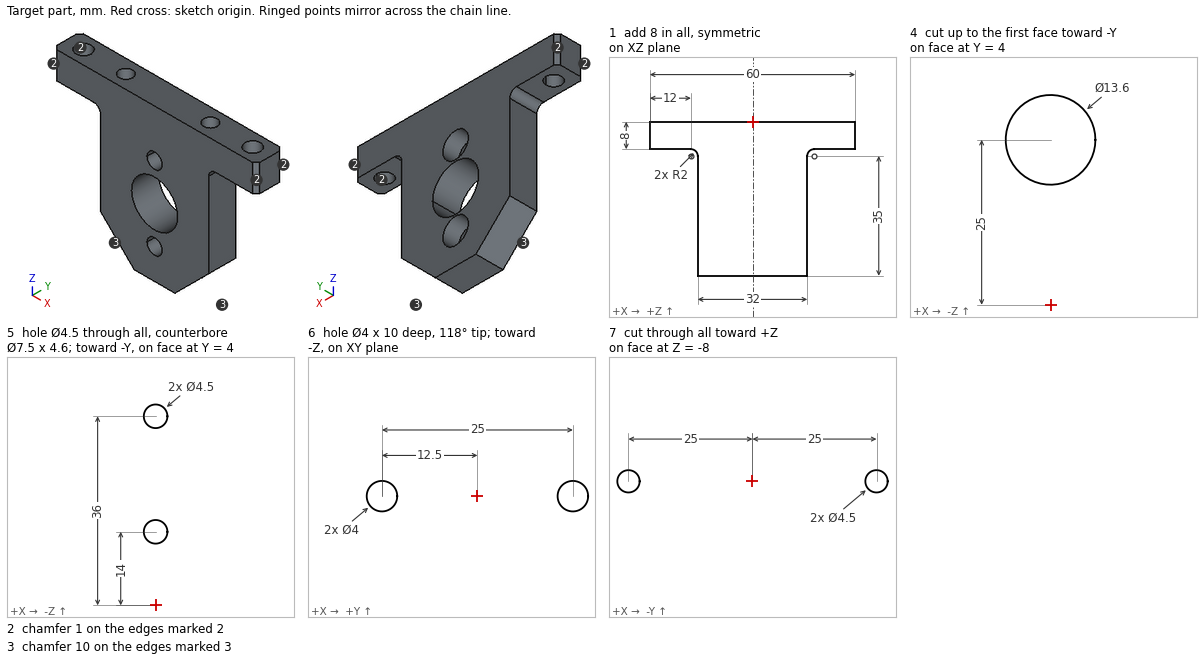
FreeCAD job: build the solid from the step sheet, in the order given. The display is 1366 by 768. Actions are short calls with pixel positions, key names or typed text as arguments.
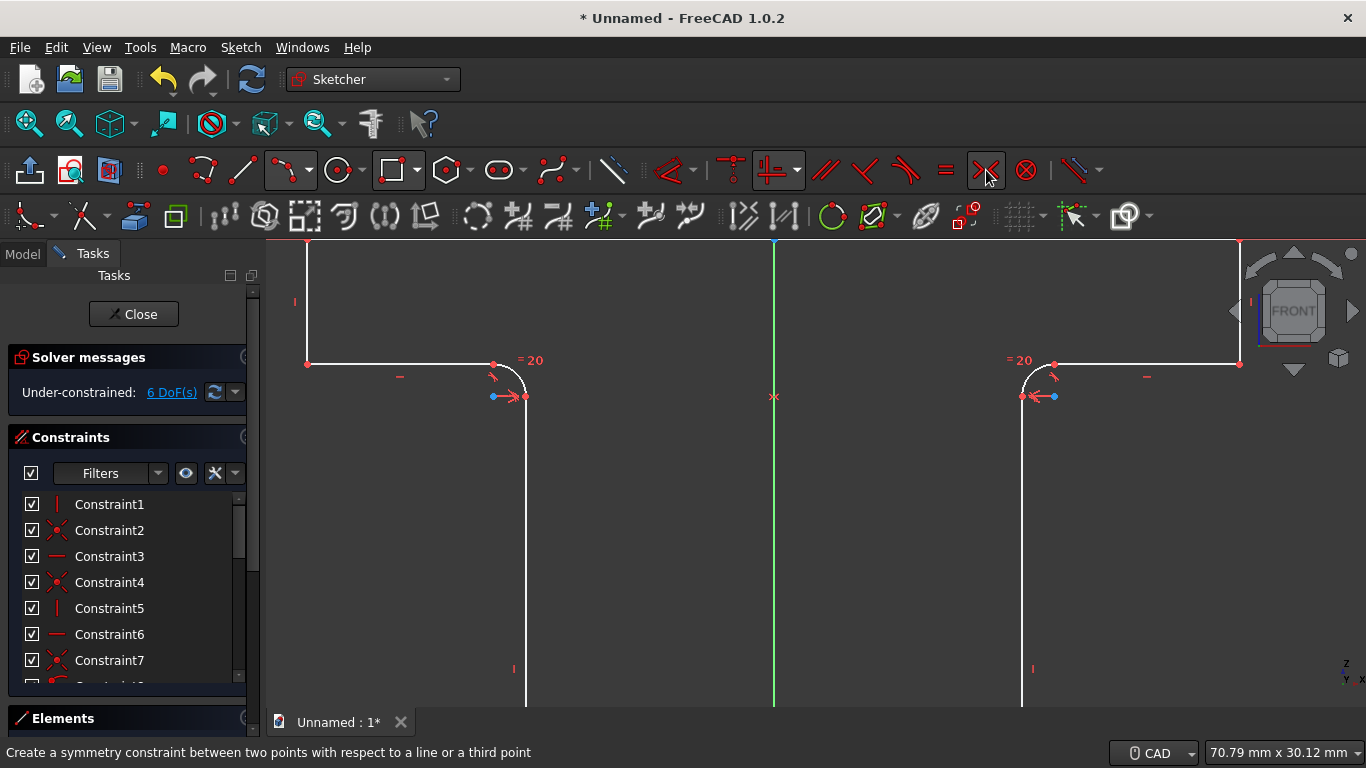
scroll(522, 382, up, 2)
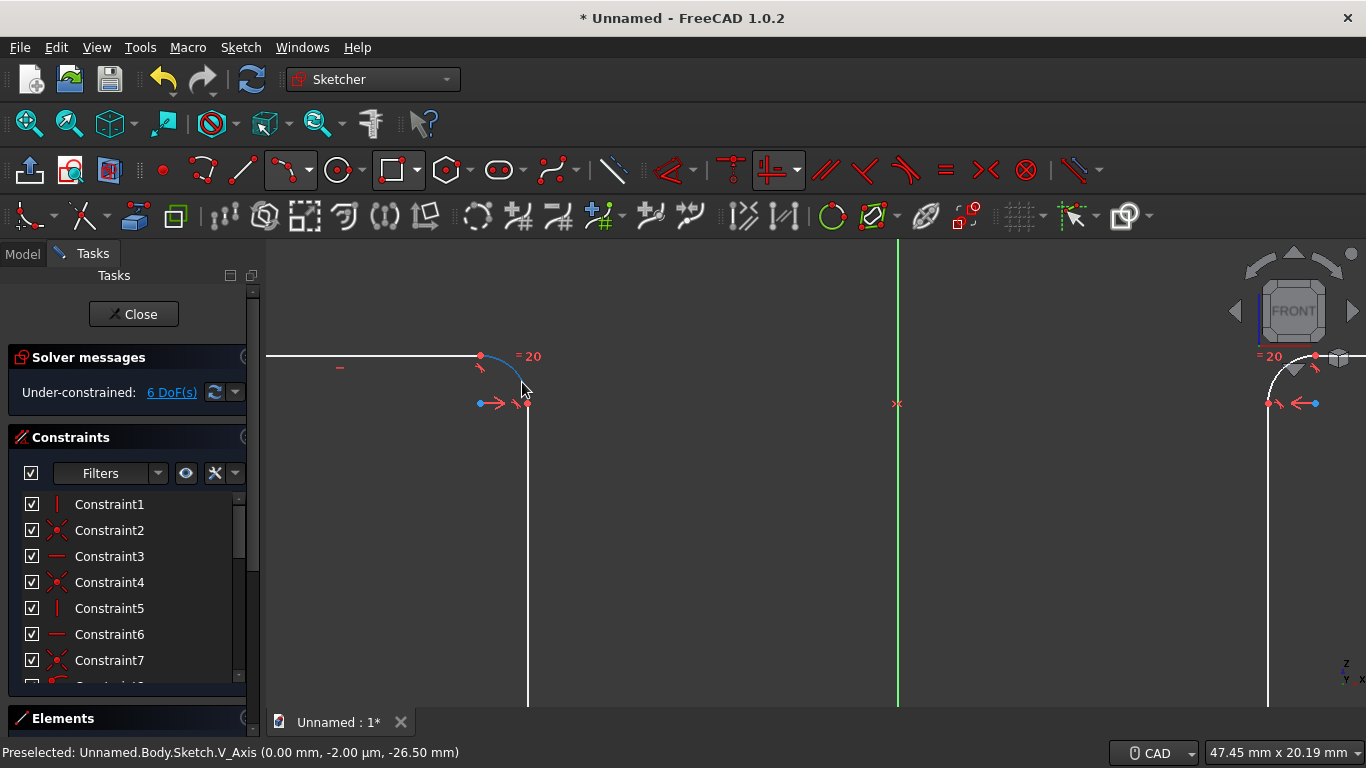
click(523, 382)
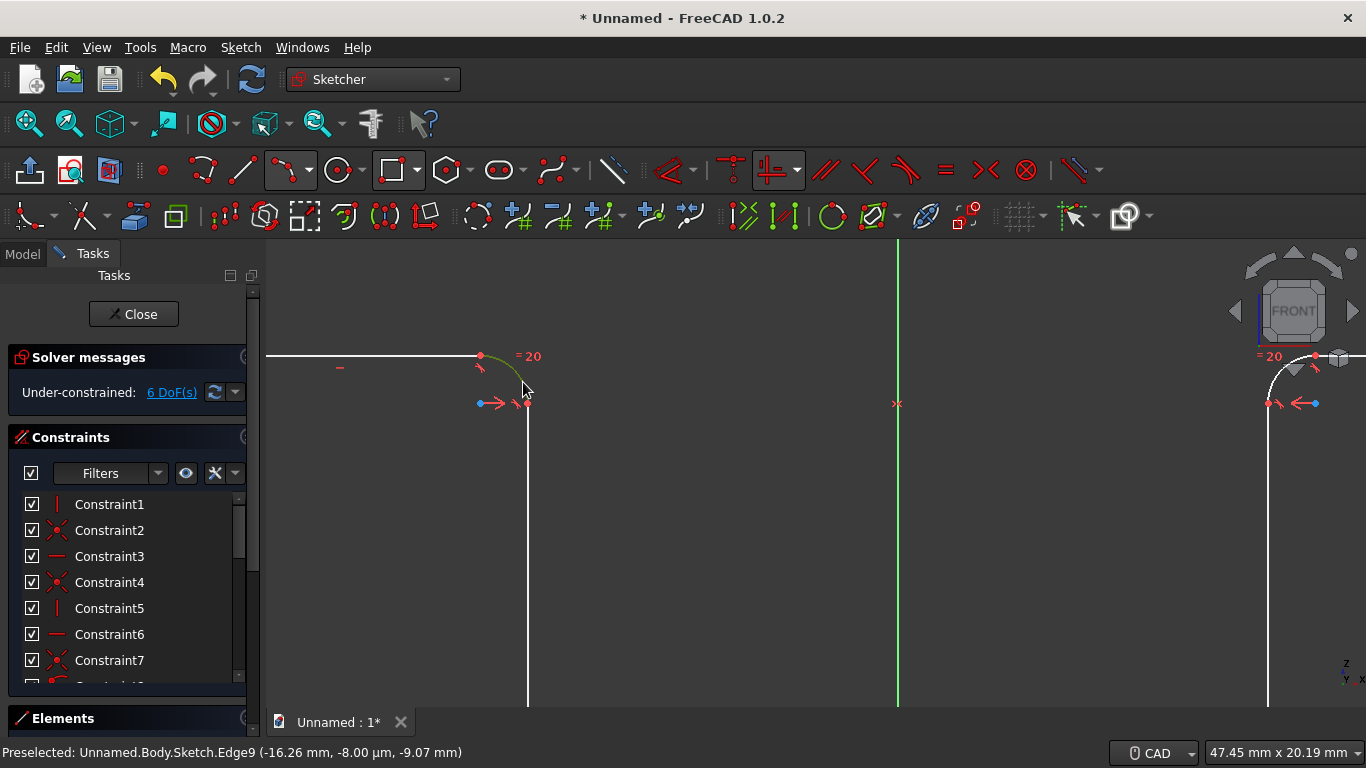
click(696, 170)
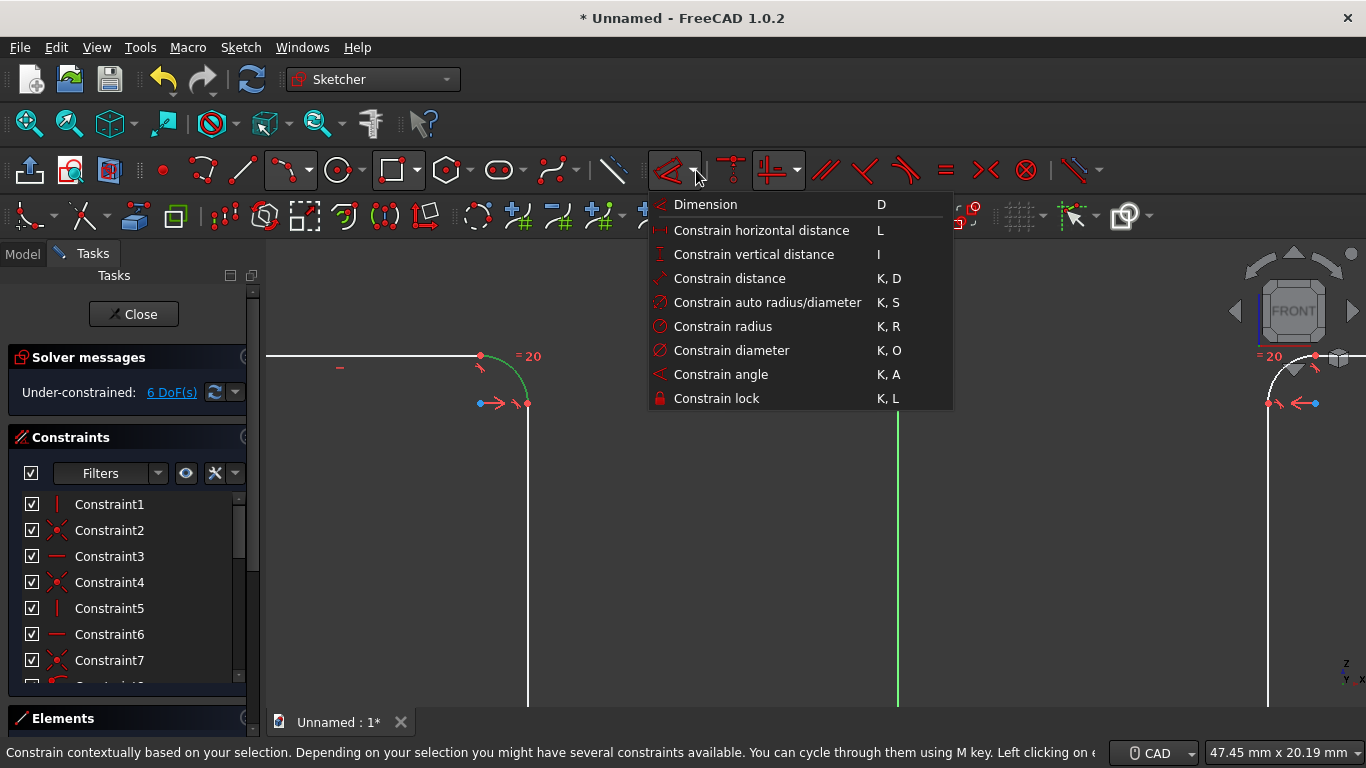
click(801, 326)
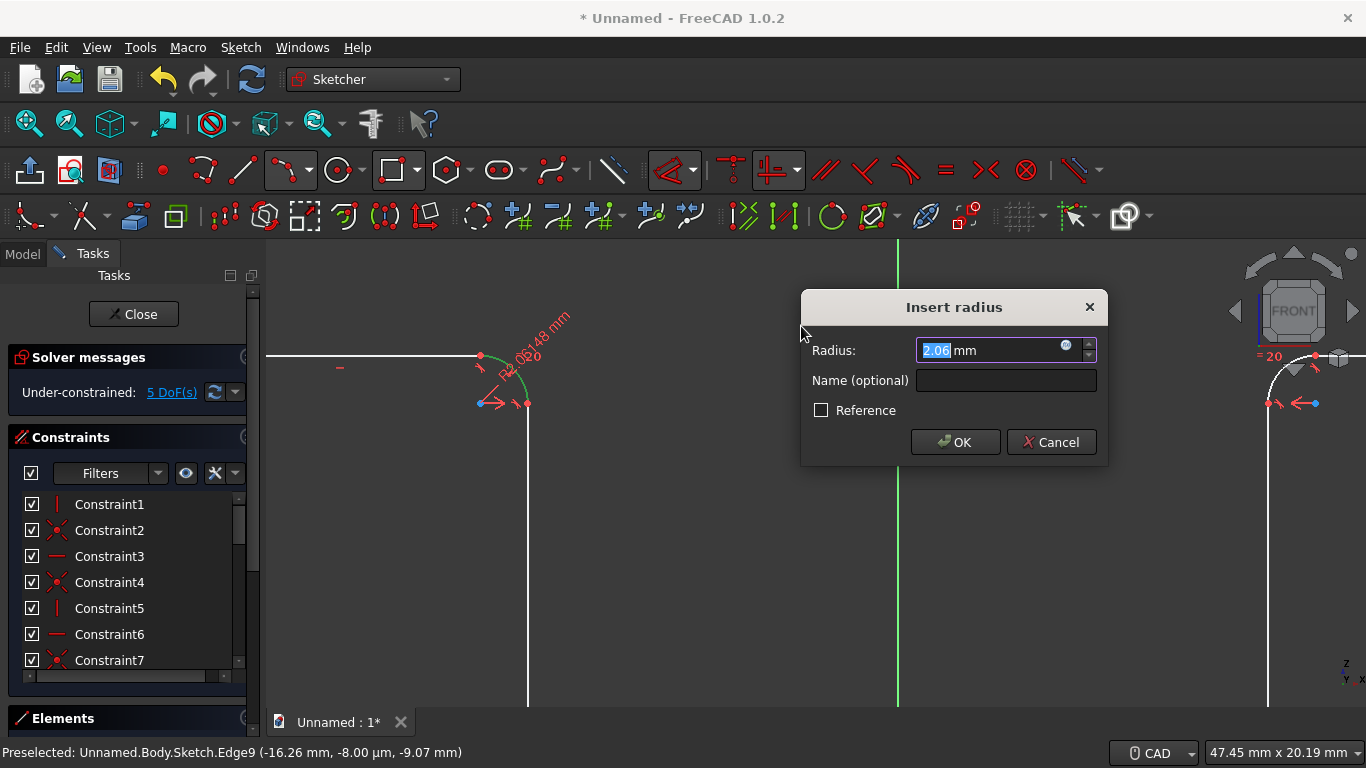
text(2)
key(Return)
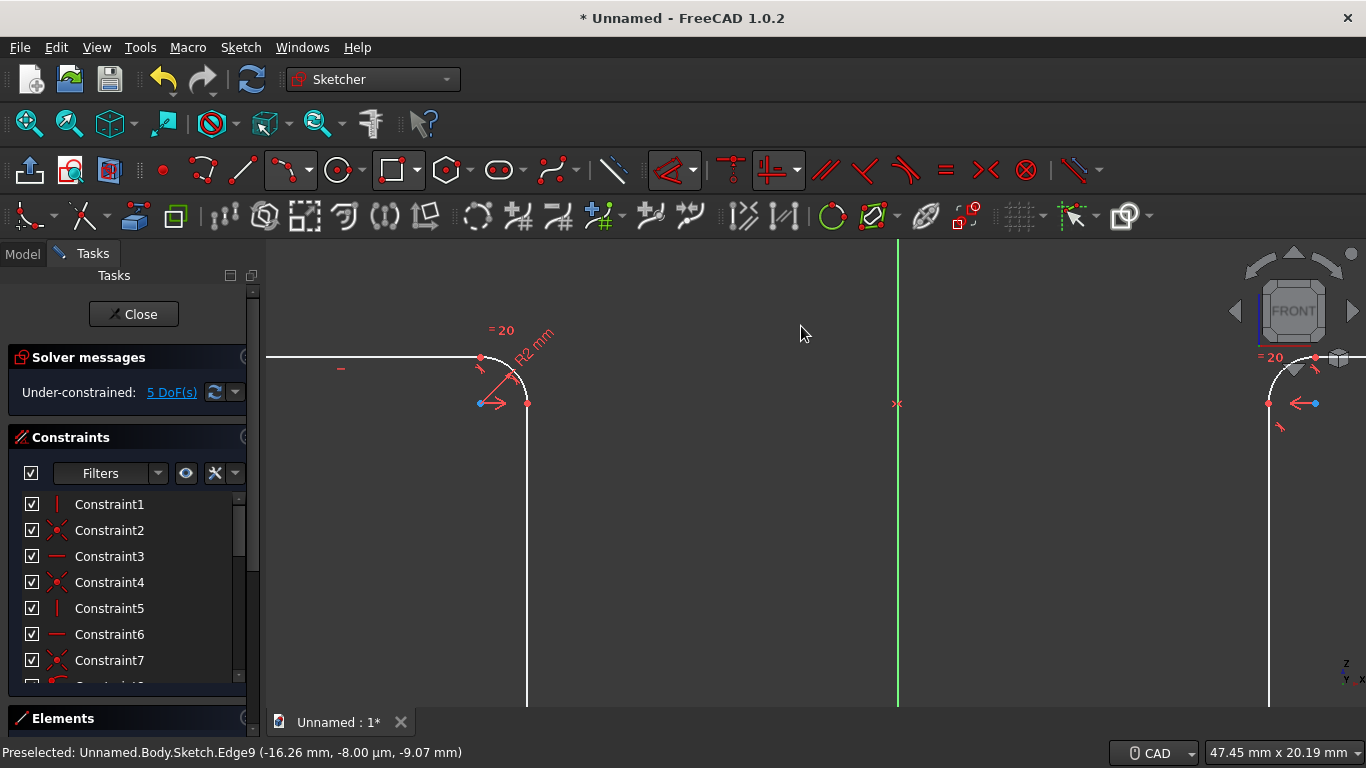
scroll(683, 379, down, 6)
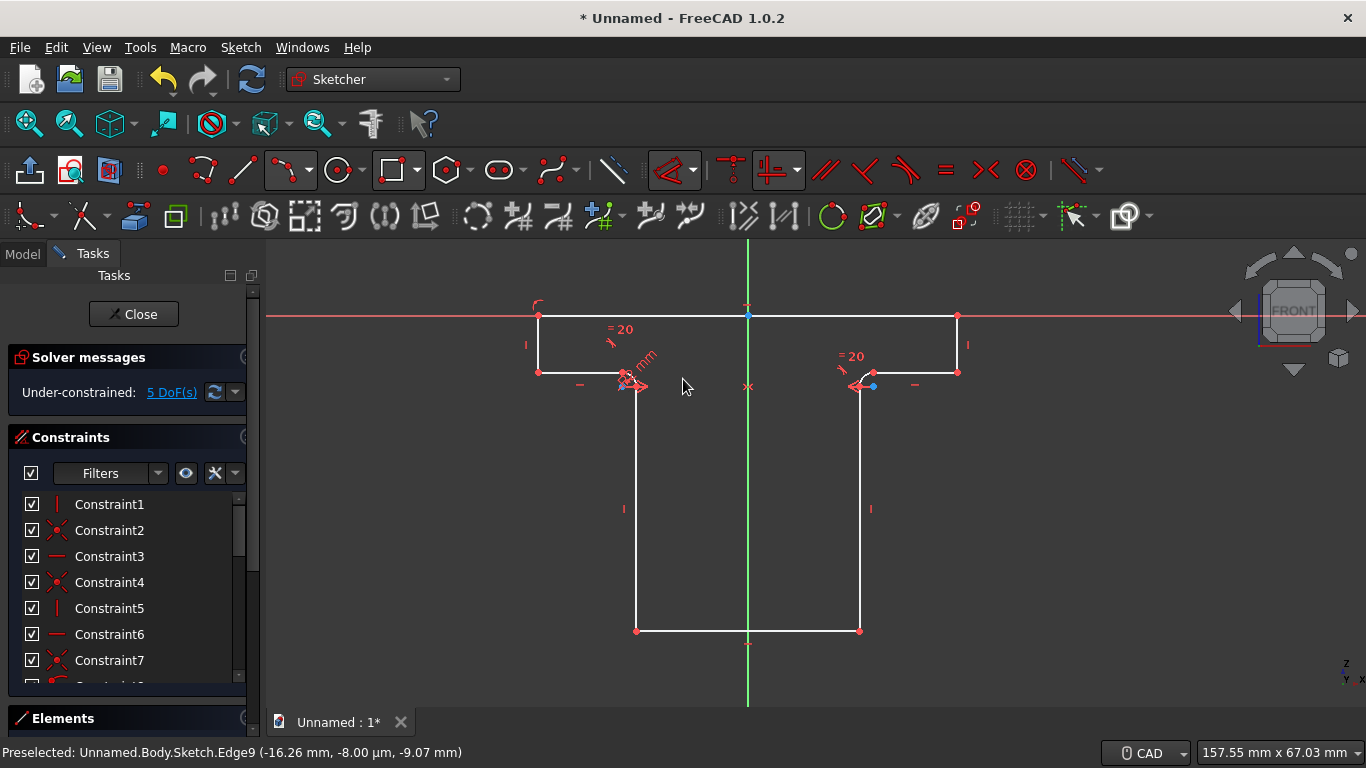
click(538, 356)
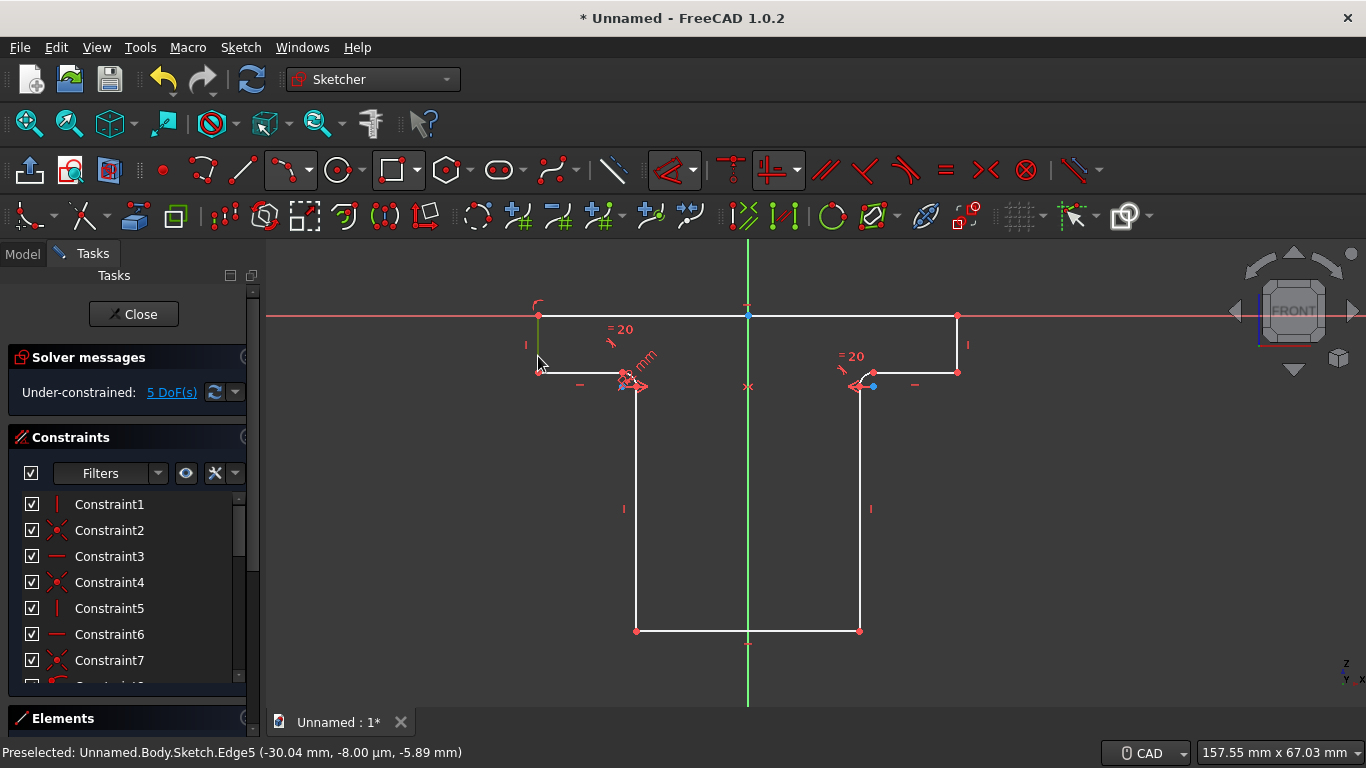
key(i)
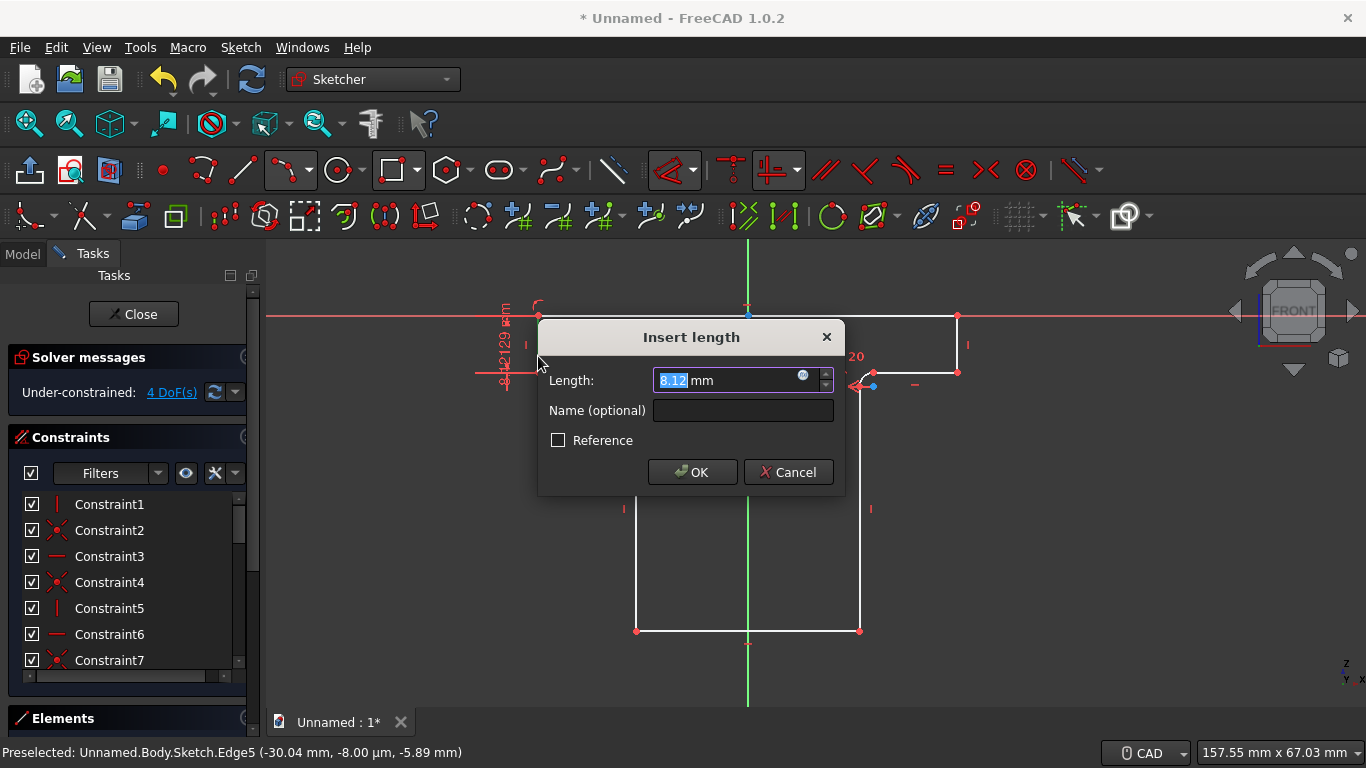
text(8)
key(Return)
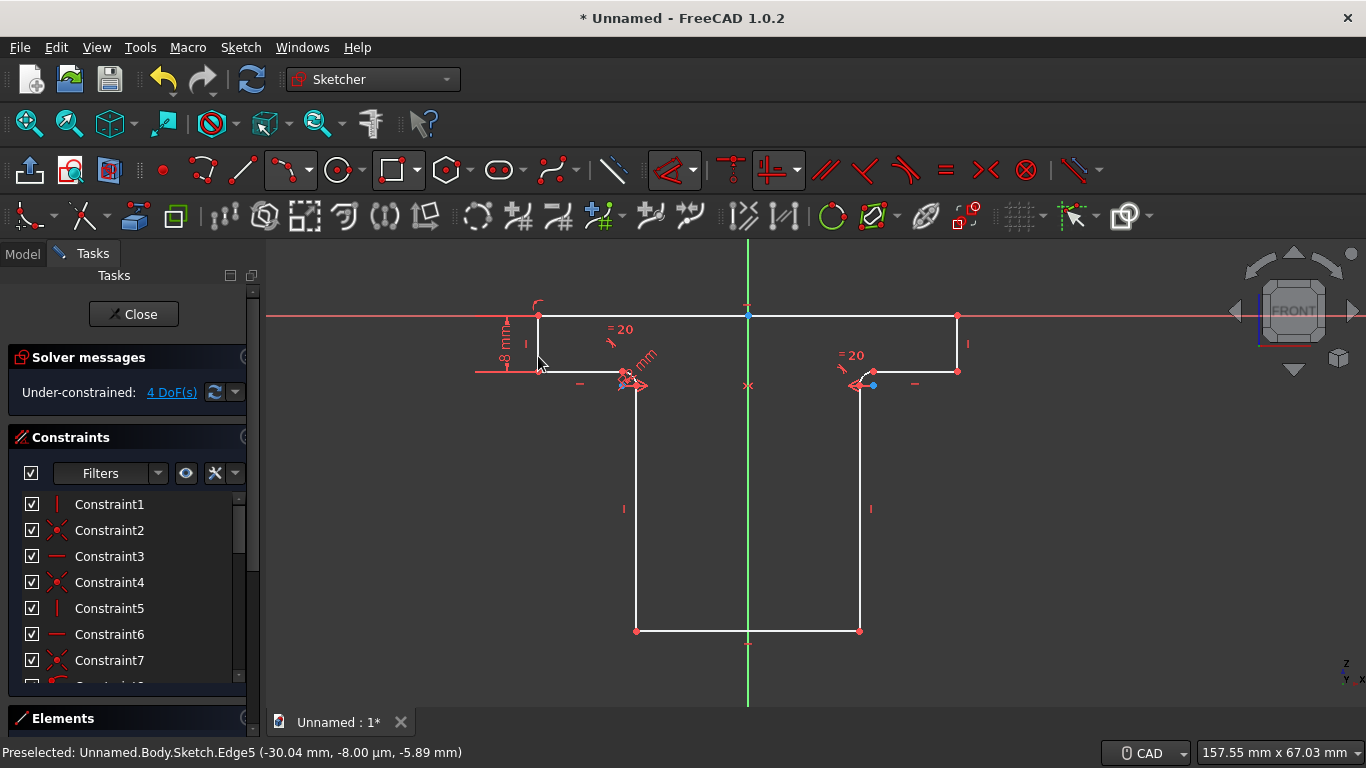
click(860, 459)